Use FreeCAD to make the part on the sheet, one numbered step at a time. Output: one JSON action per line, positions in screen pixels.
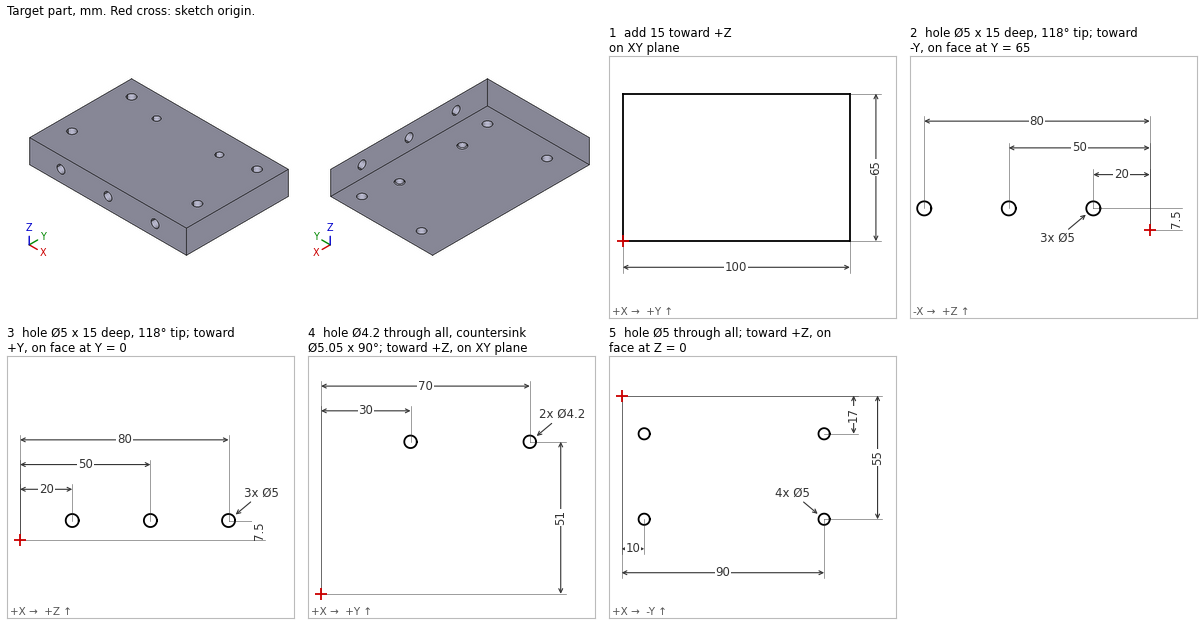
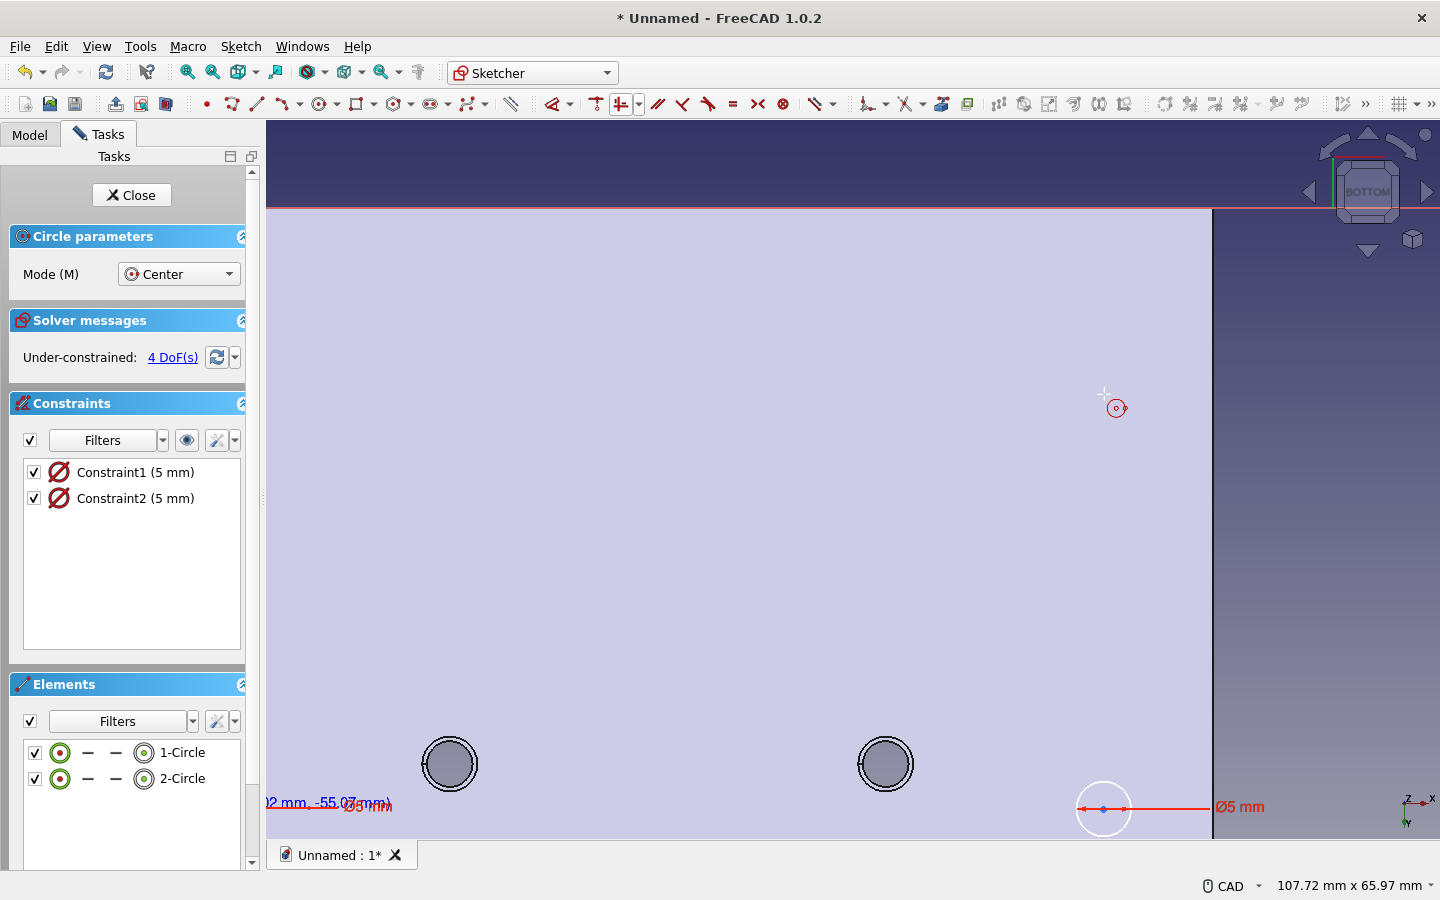
{"action": "left_click", "coordinate": [1104, 393]}
{"action": "mouse_move", "coordinate": [1123, 374]}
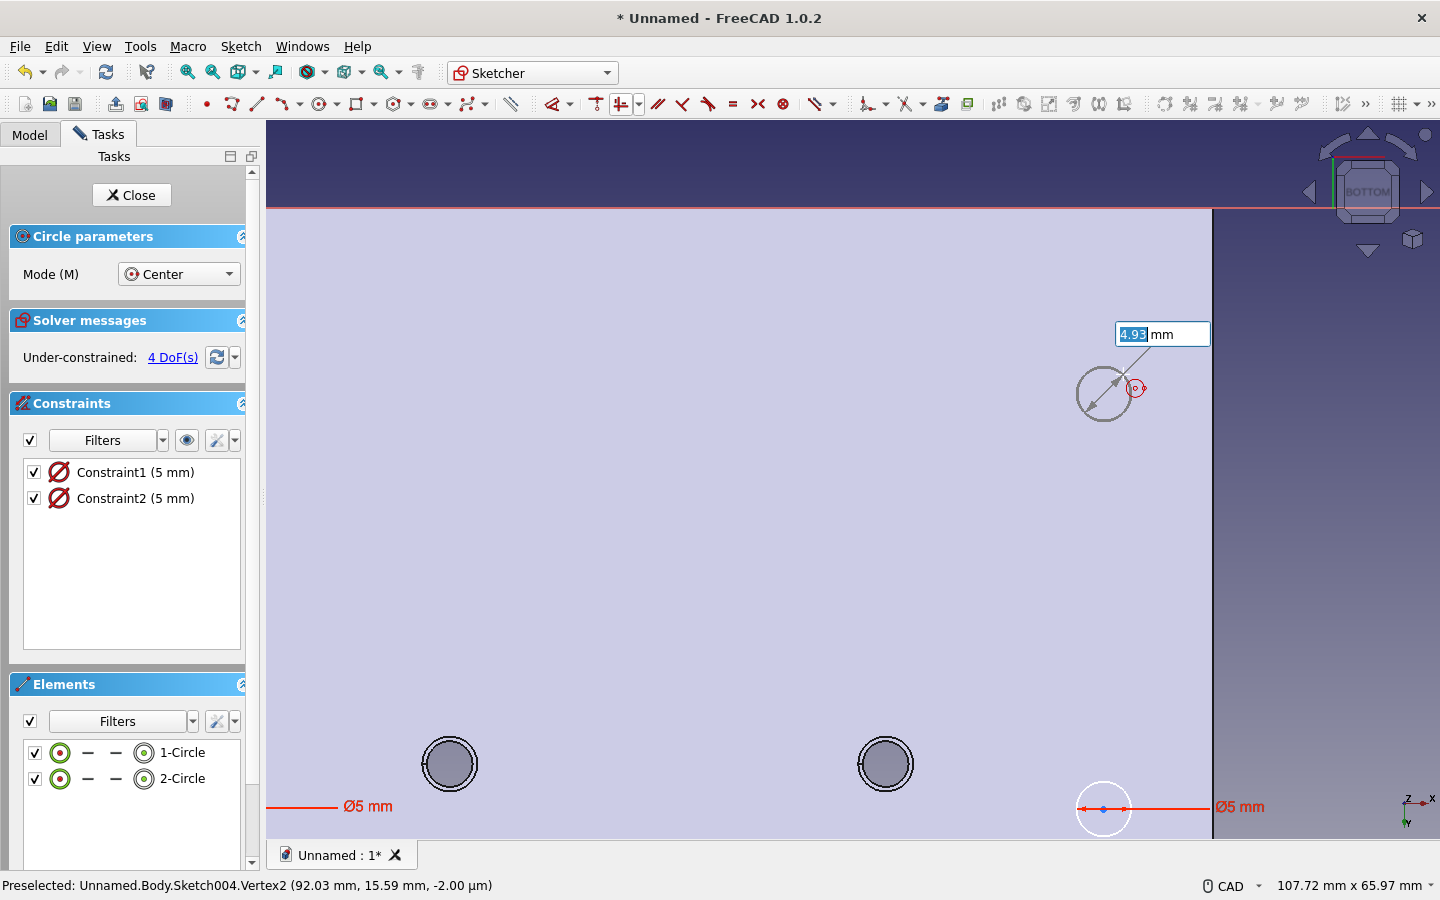
{"action": "type", "text": "5"}
{"action": "key", "text": "Return"}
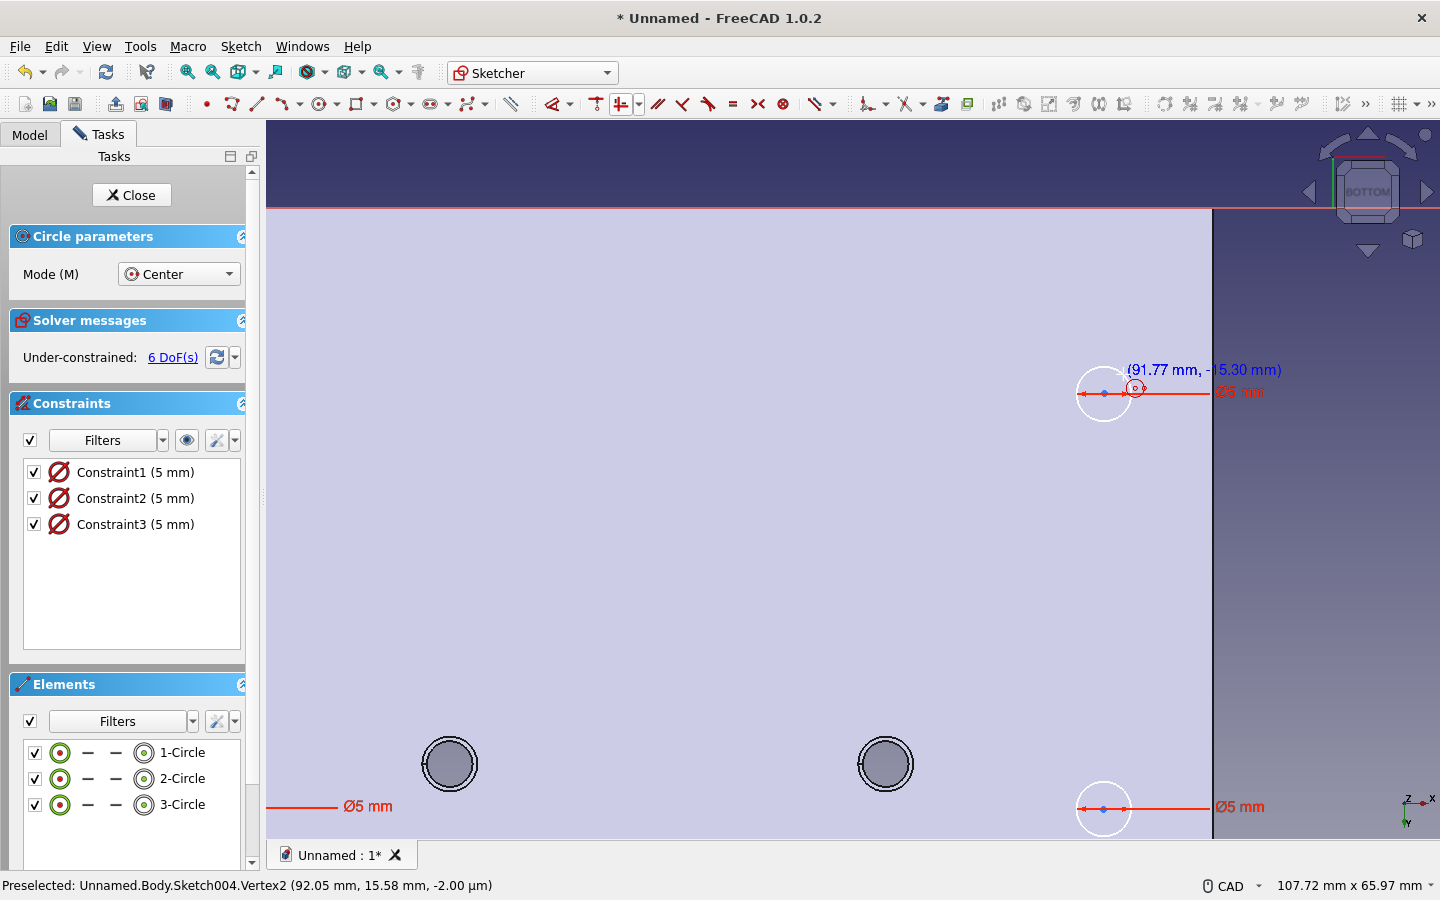
{"action": "scroll", "coordinate": [1105, 394], "scroll_direction": "down", "scroll_amount": 2}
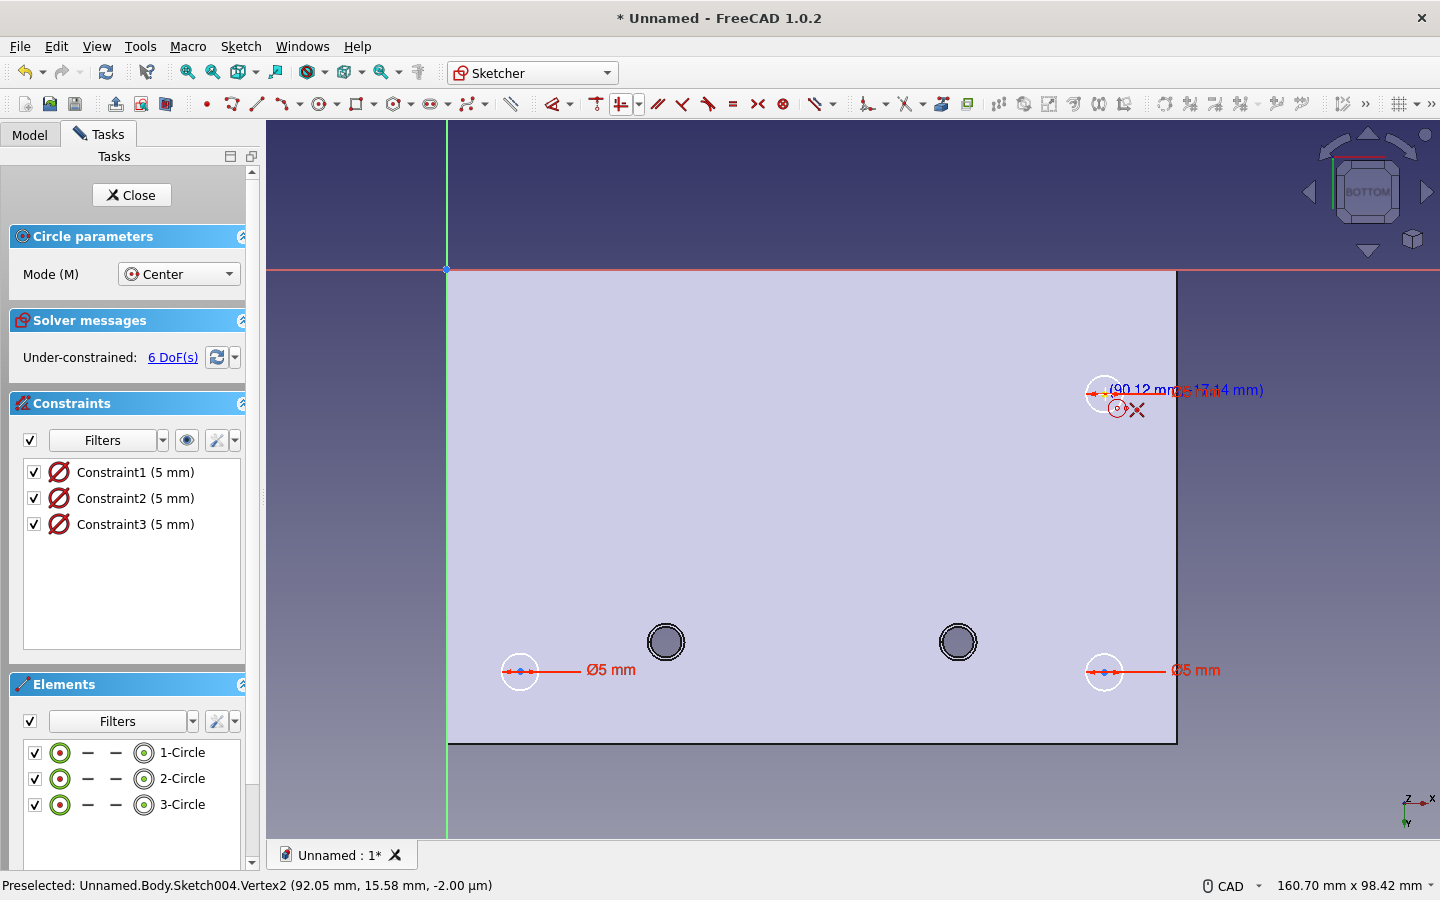
{"action": "scroll", "coordinate": [520, 394], "scroll_direction": "up", "scroll_amount": 2}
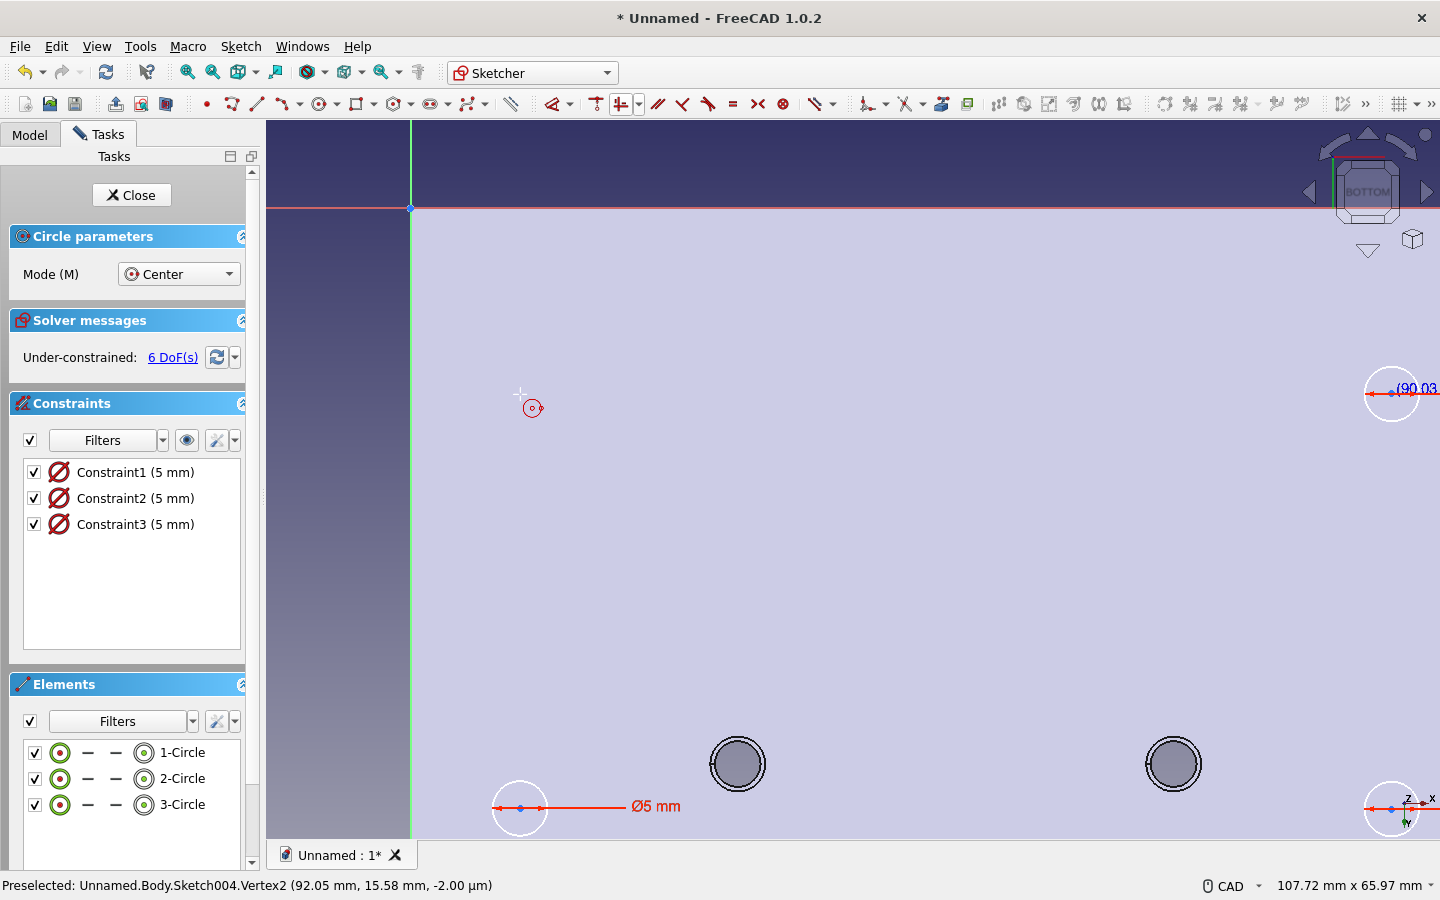
{"action": "left_click", "coordinate": [520, 393]}
{"action": "mouse_move", "coordinate": [539, 374]}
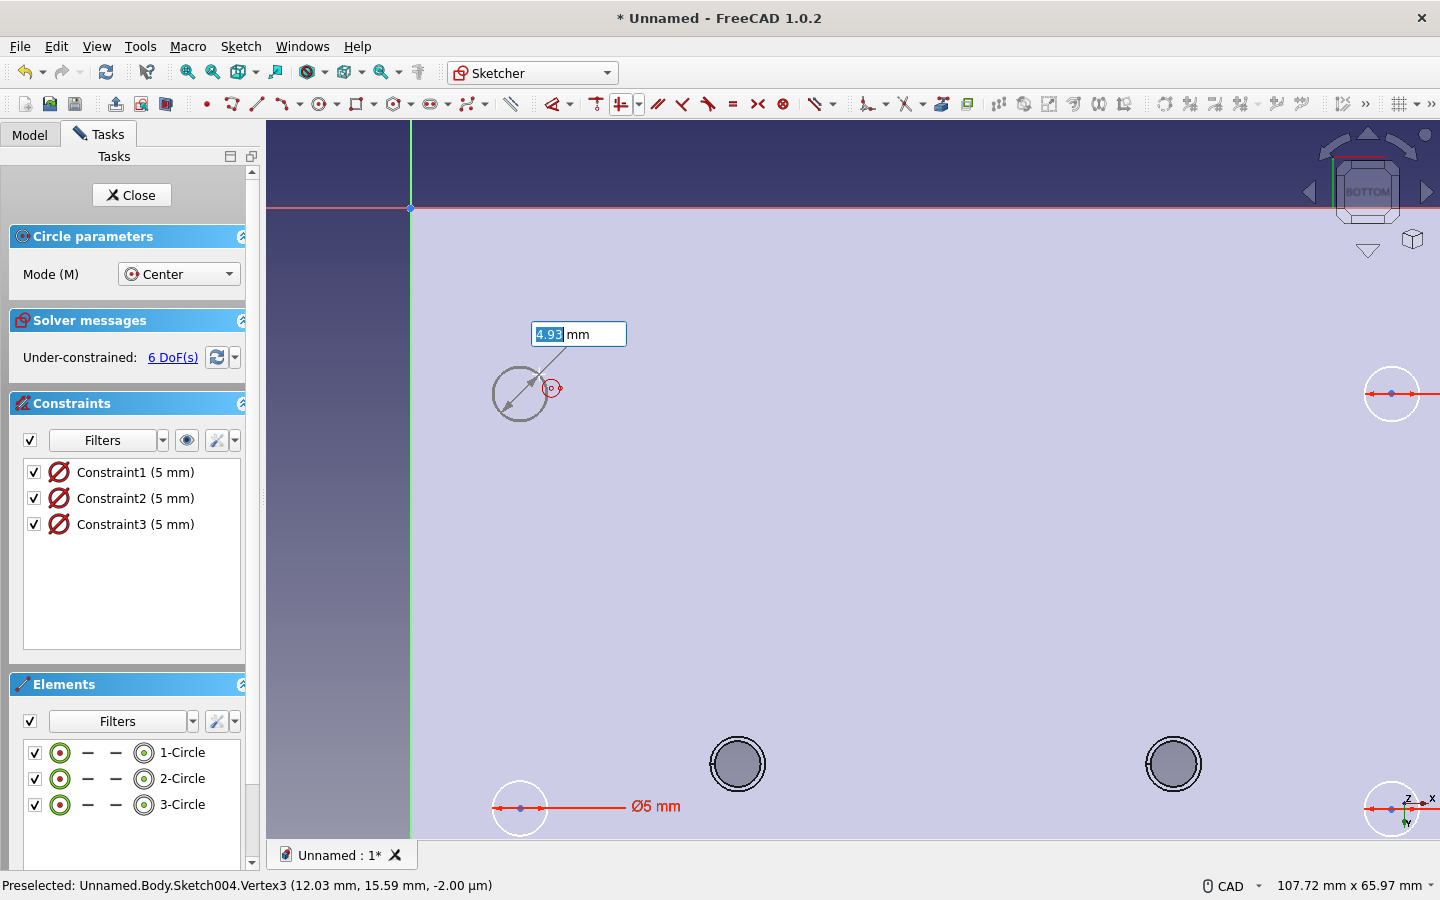
{"action": "type", "text": "5"}
{"action": "key", "text": "Return"}
{"action": "key", "text": "Escape"}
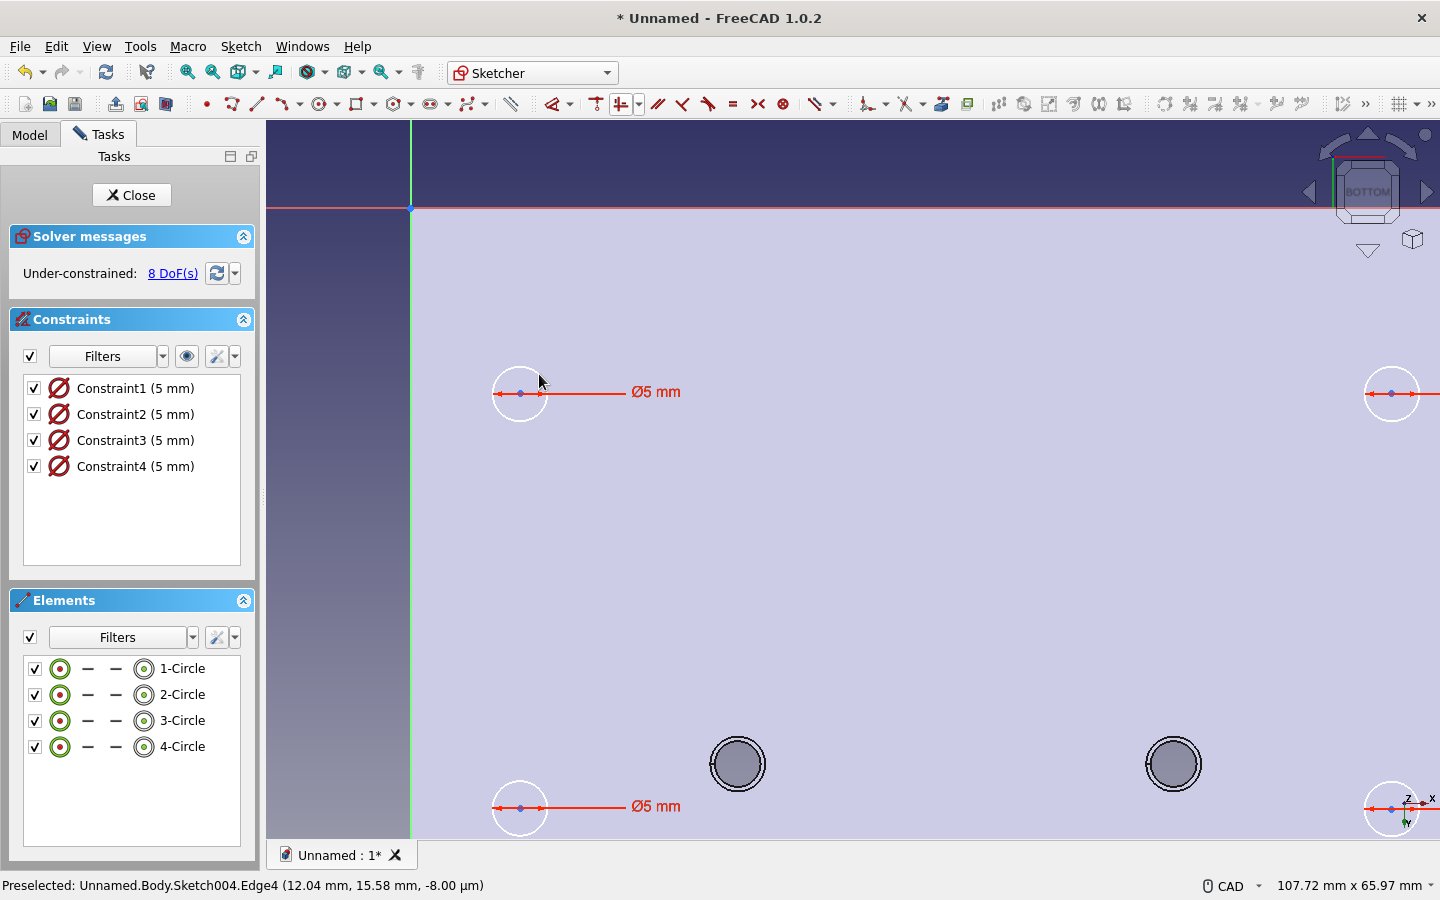
{"action": "scroll", "coordinate": [519, 394], "scroll_direction": "down", "scroll_amount": 2}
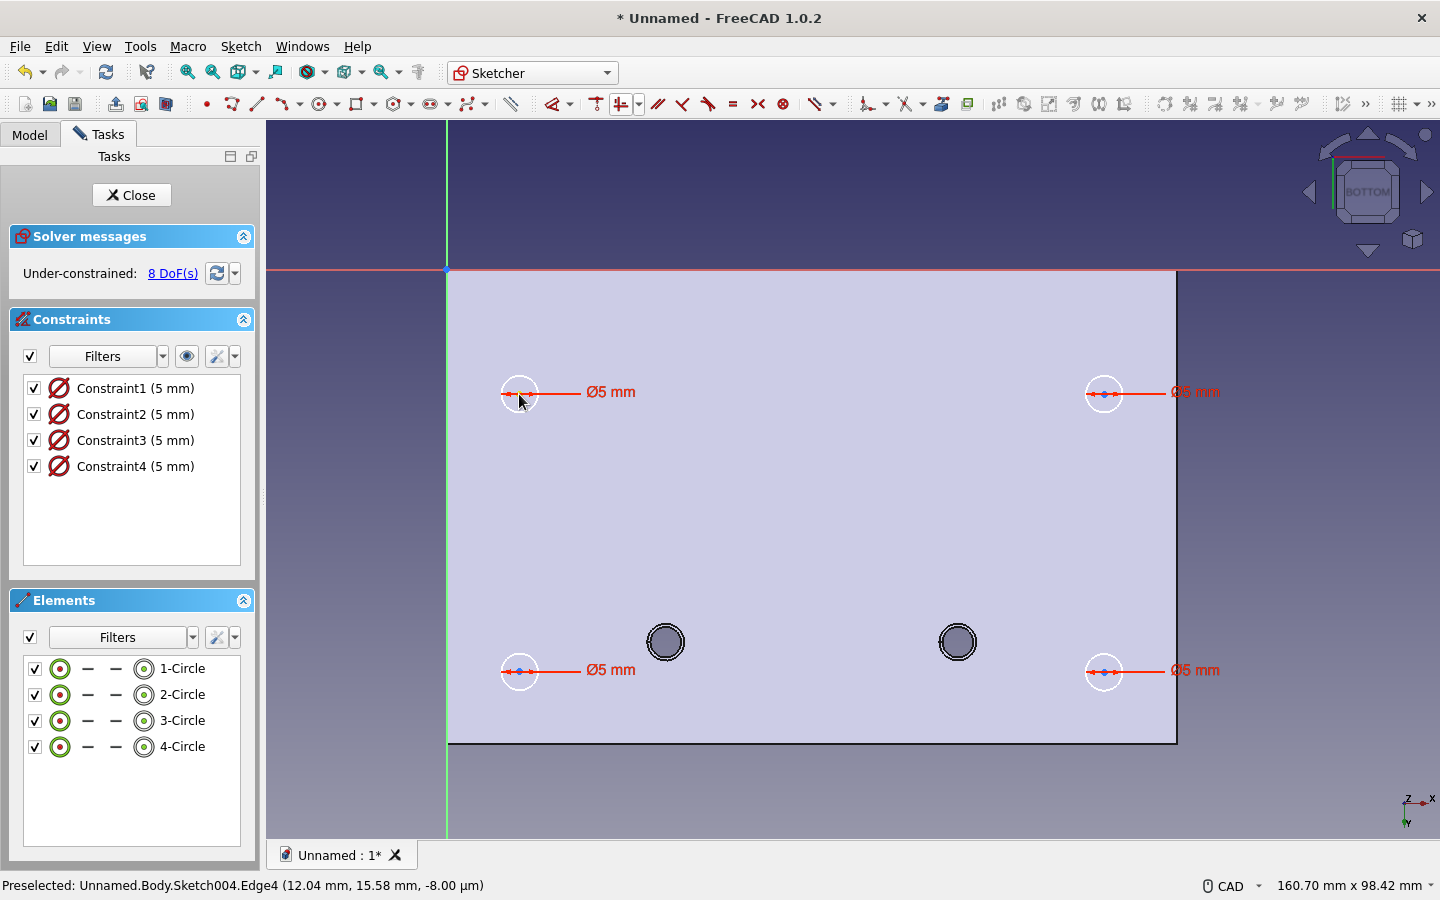
{"action": "left_click", "coordinate": [1104, 672]}